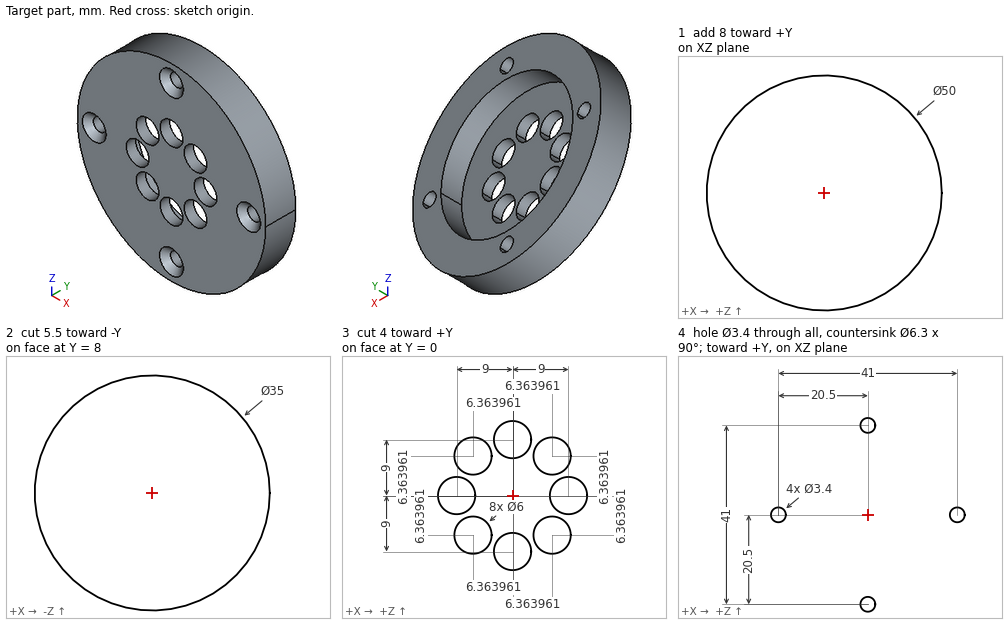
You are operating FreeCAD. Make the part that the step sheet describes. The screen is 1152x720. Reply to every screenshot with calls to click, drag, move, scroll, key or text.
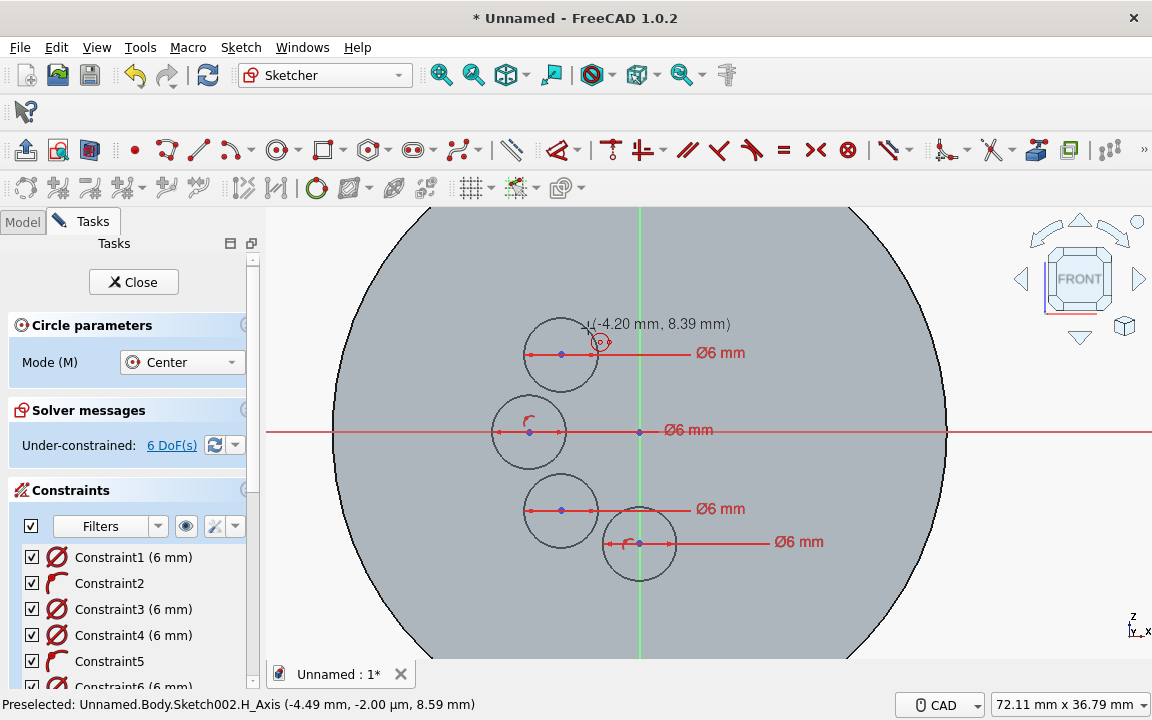
click(640, 322)
move(666, 295)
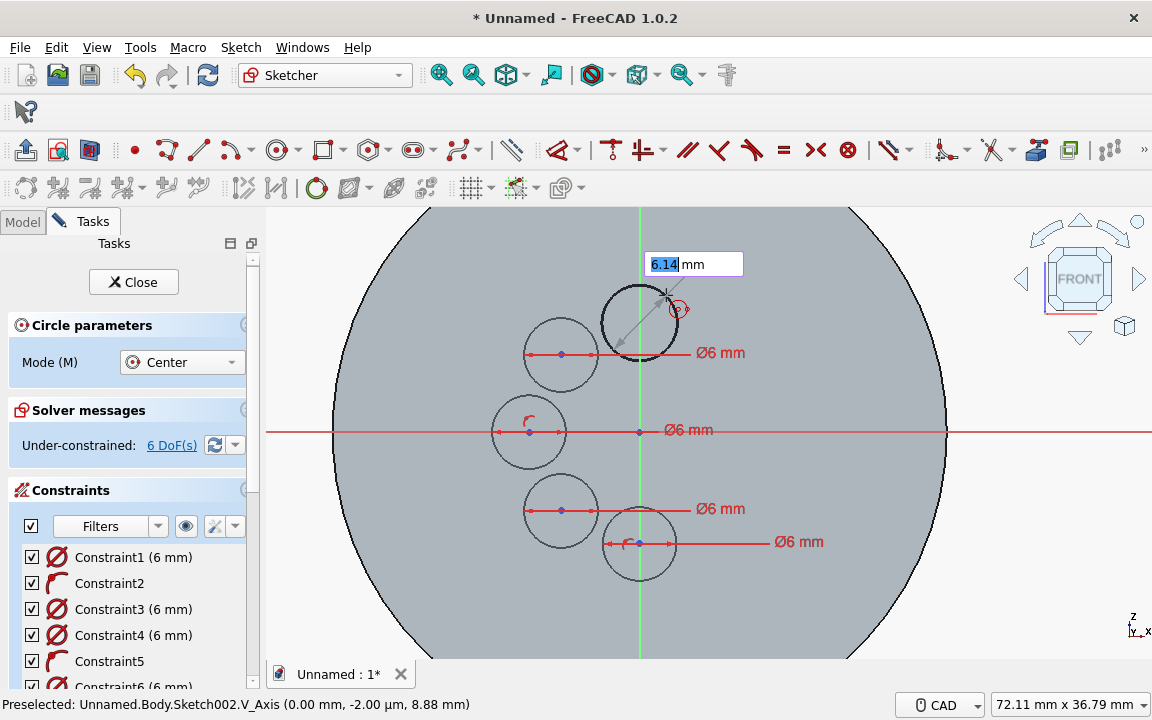
text(6)
key(Return)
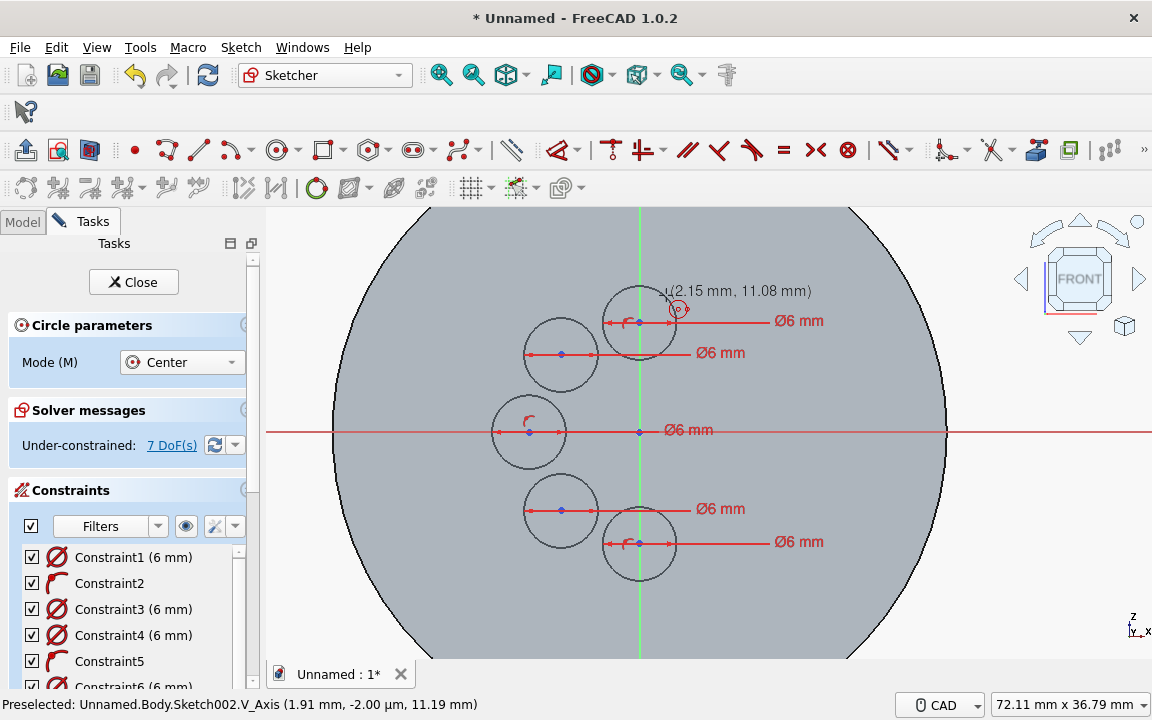
click(718, 354)
move(744, 328)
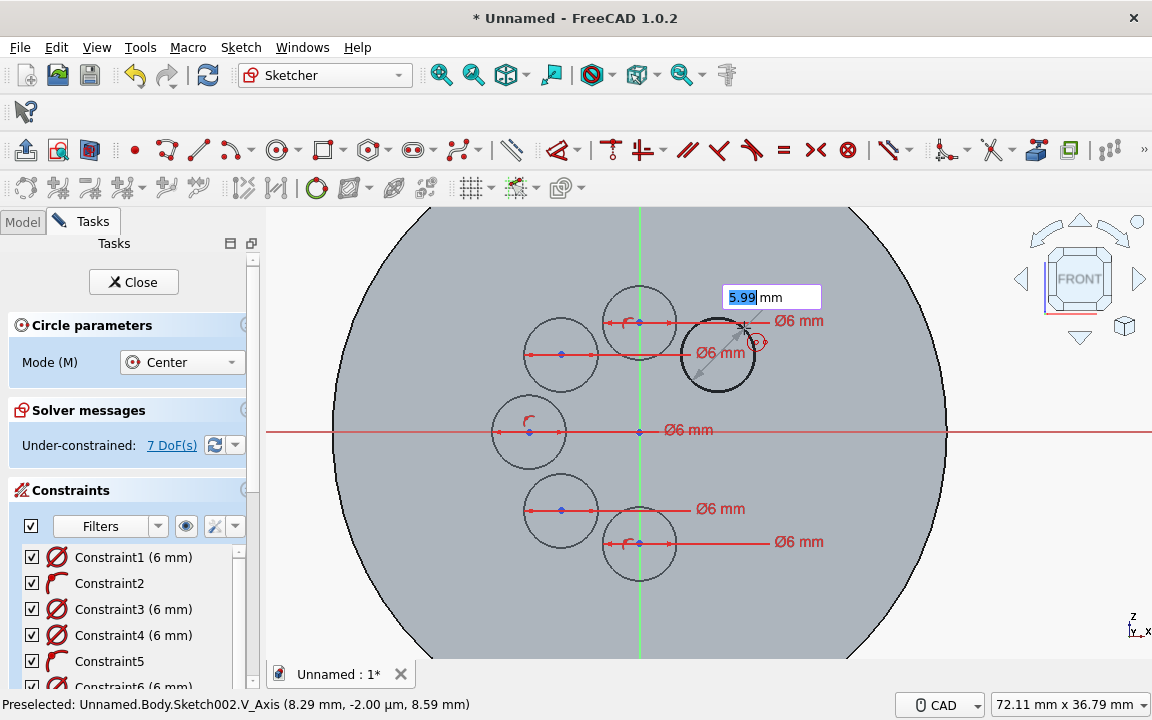
text(6)
key(Return)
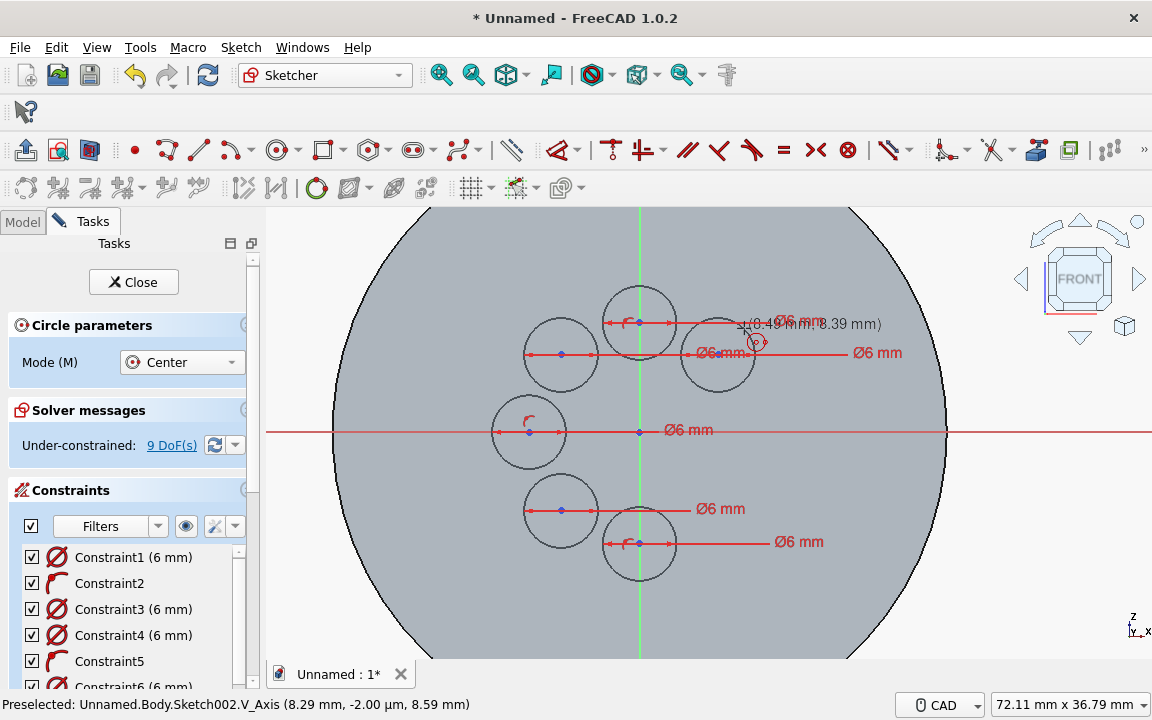
click(750, 432)
move(776, 406)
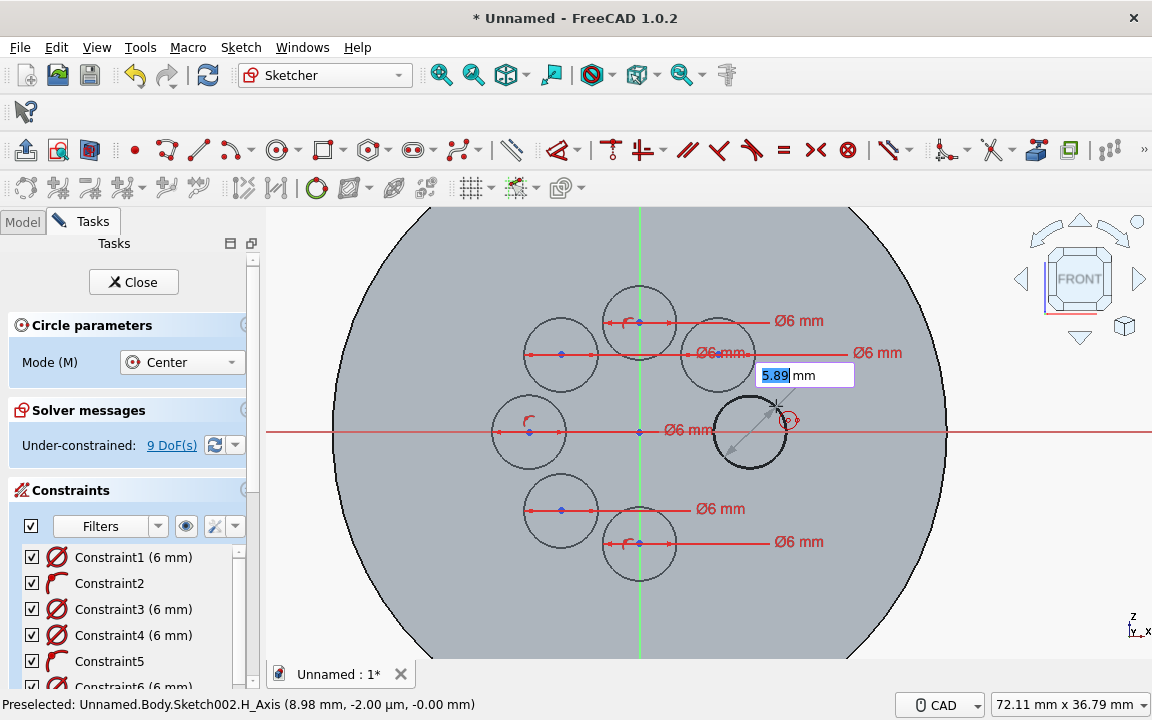
text(6)
key(Return)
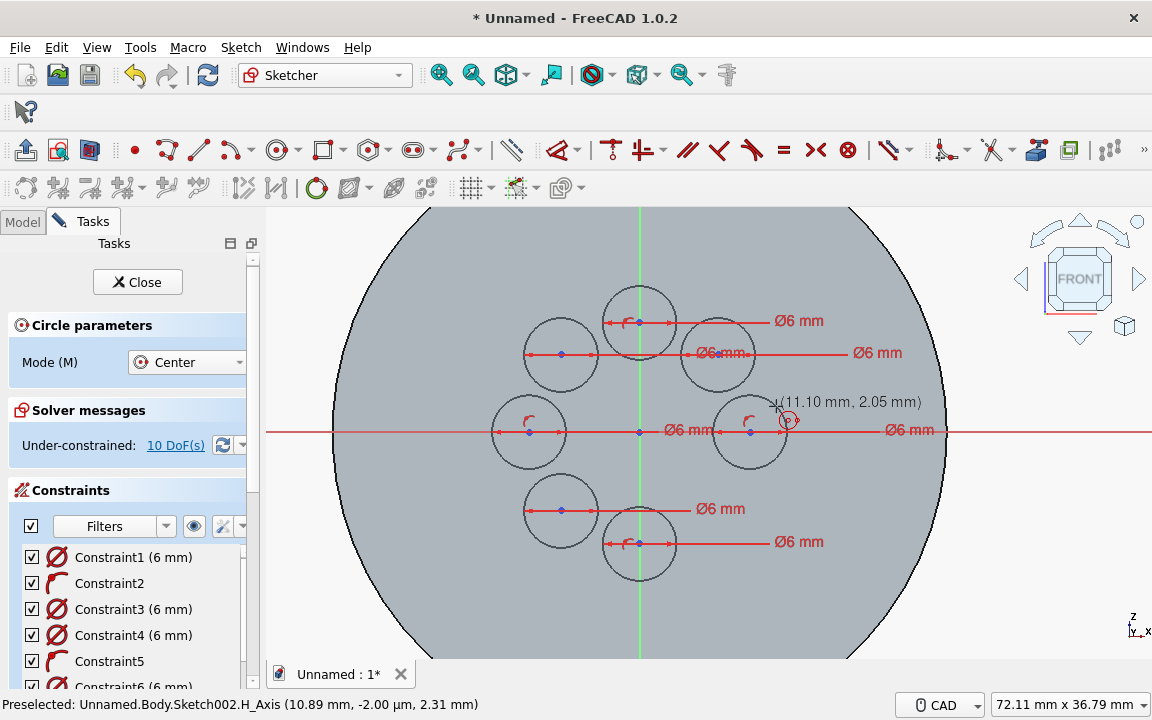
click(718, 510)
move(744, 484)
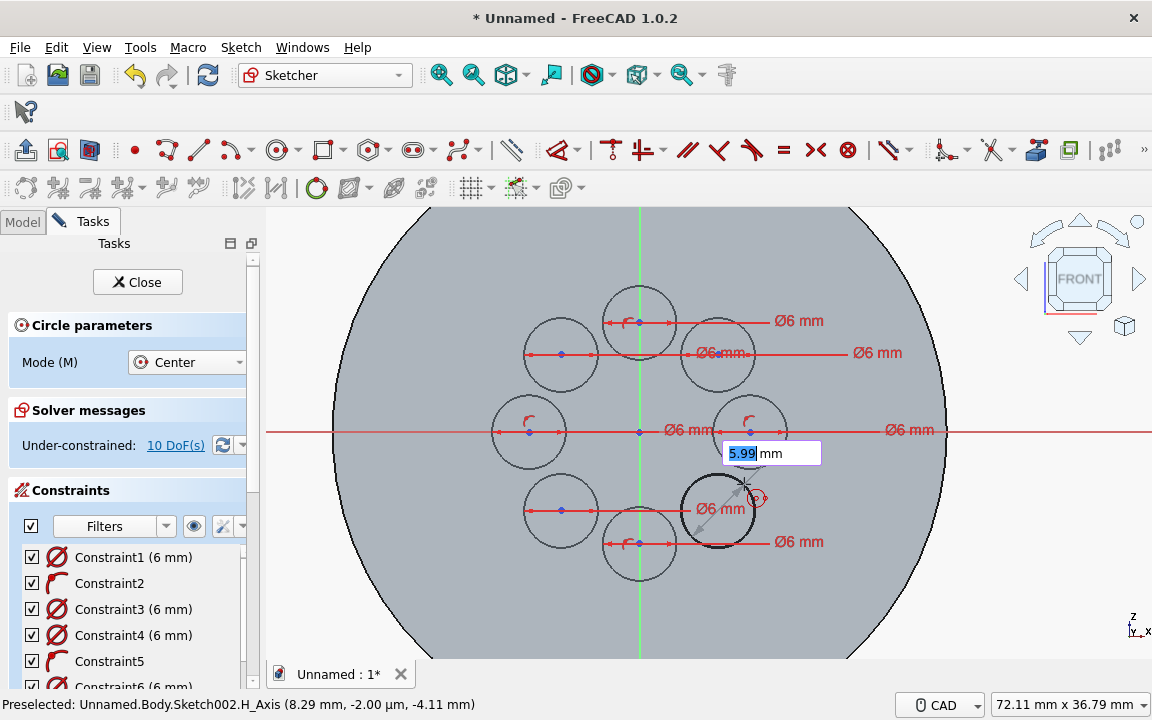
text(6)
key(Return)
key(Escape)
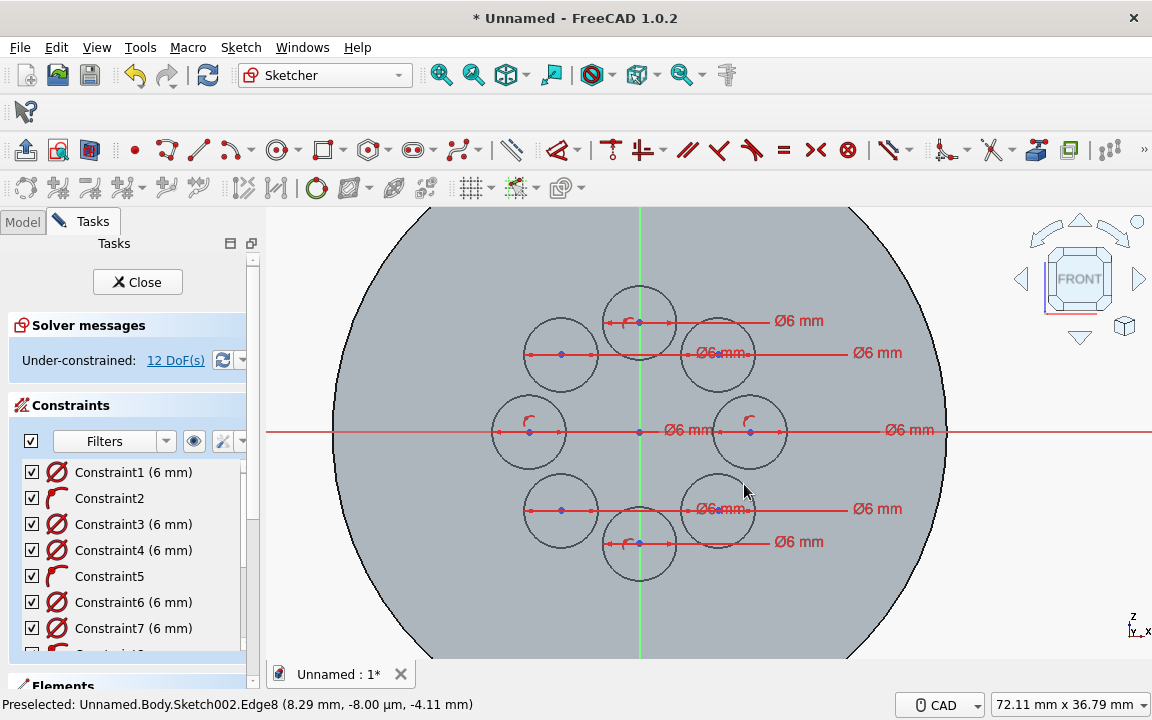
click(558, 150)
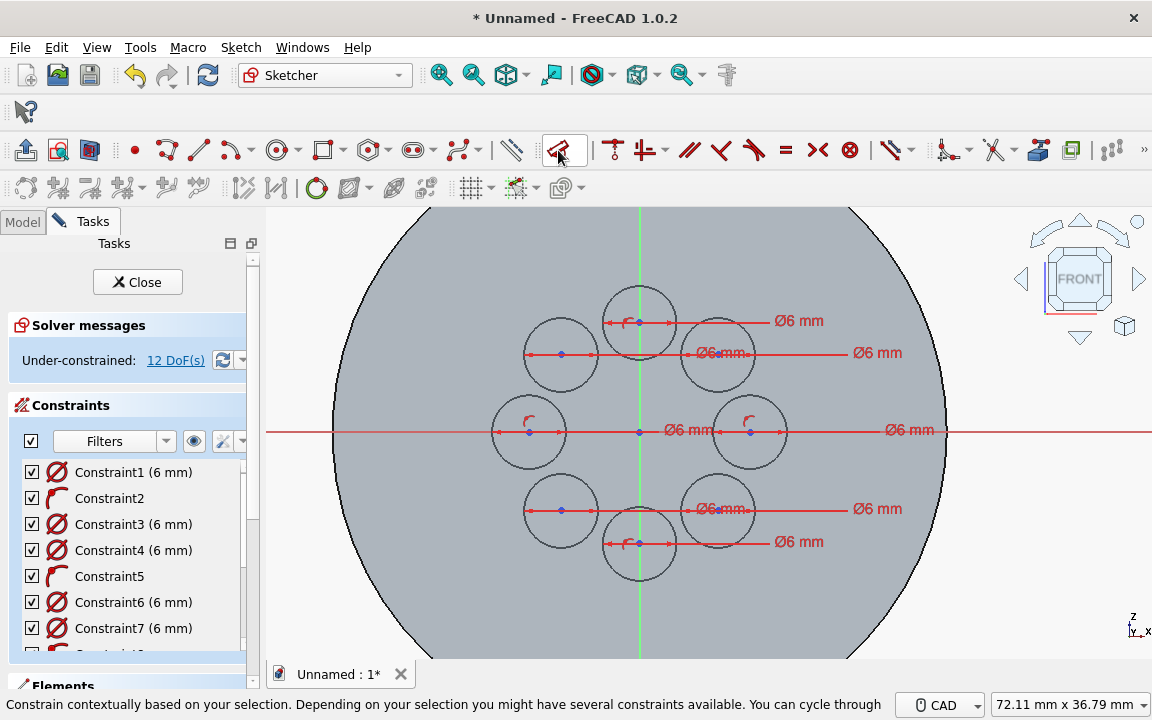
click(640, 544)
click(674, 488)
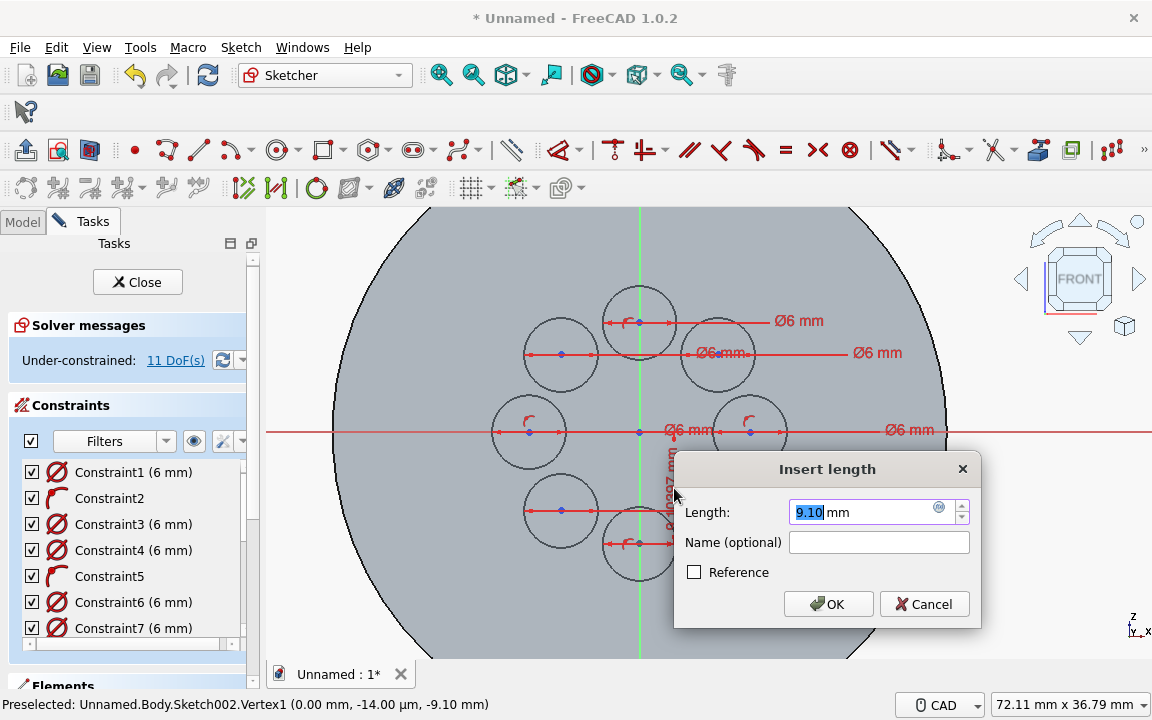
text(9)
key(Return)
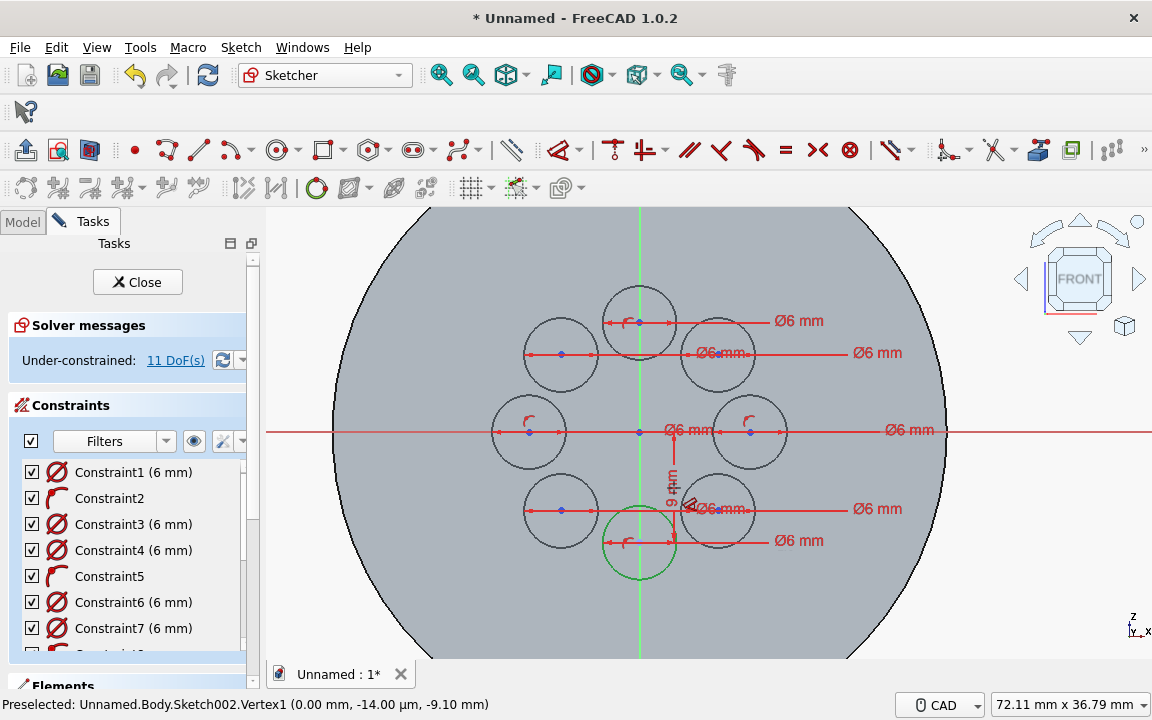
click(529, 432)
click(584, 466)